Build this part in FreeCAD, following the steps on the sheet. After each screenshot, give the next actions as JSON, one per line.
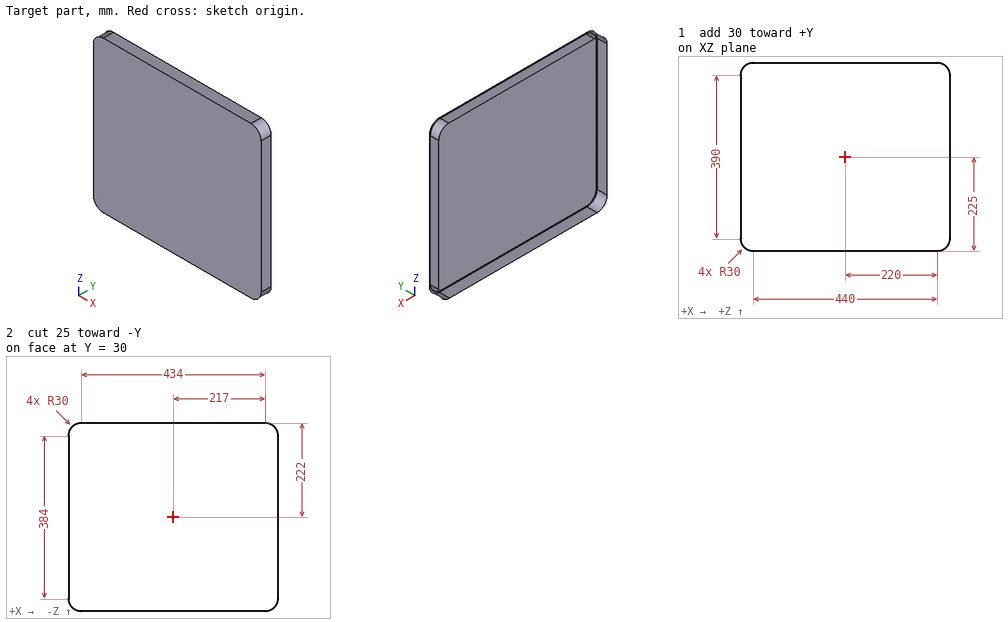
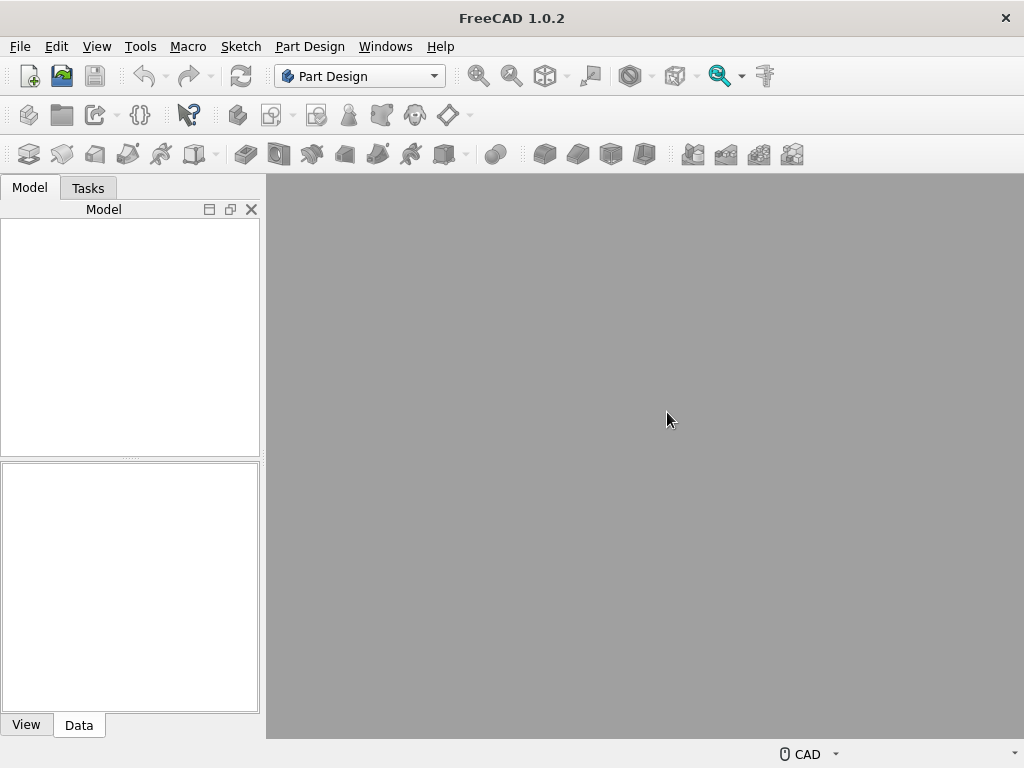
{"action": "left_click", "coordinate": [29, 76]}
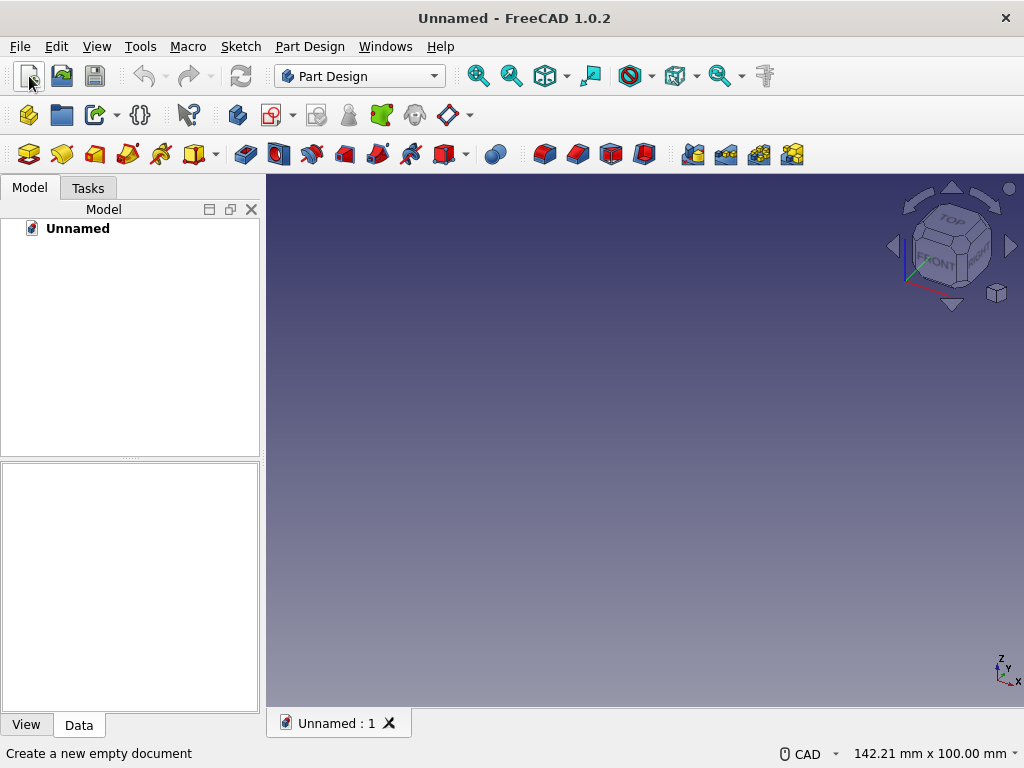
{"action": "left_click", "coordinate": [270, 116]}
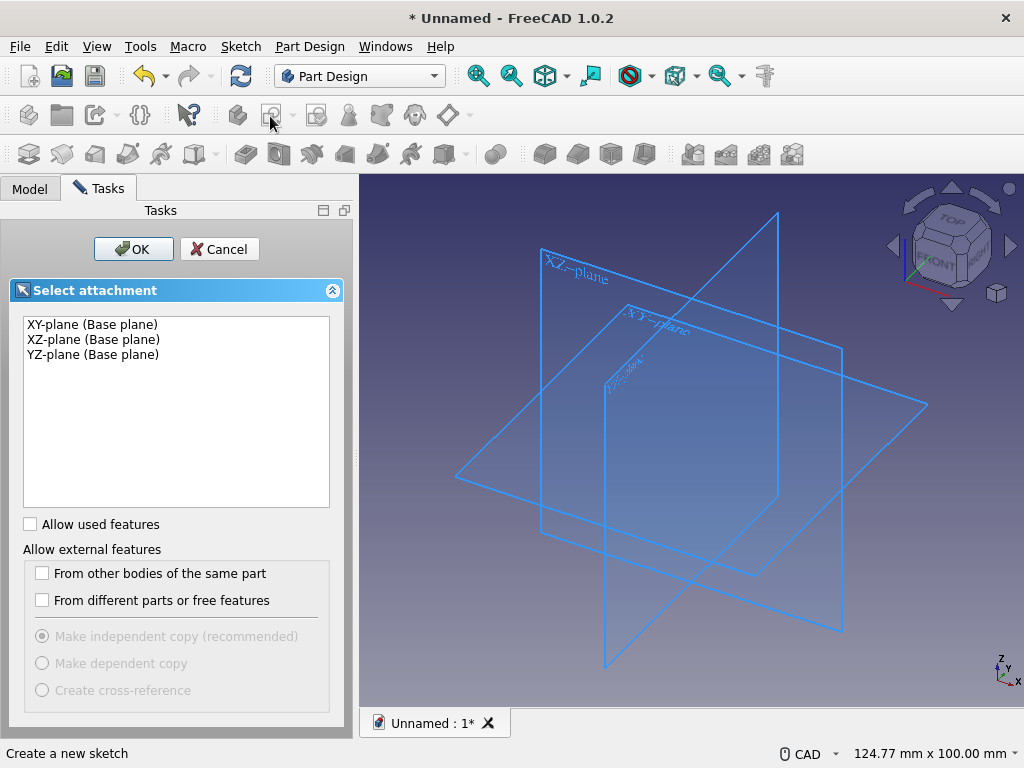
{"action": "left_click", "coordinate": [84, 340]}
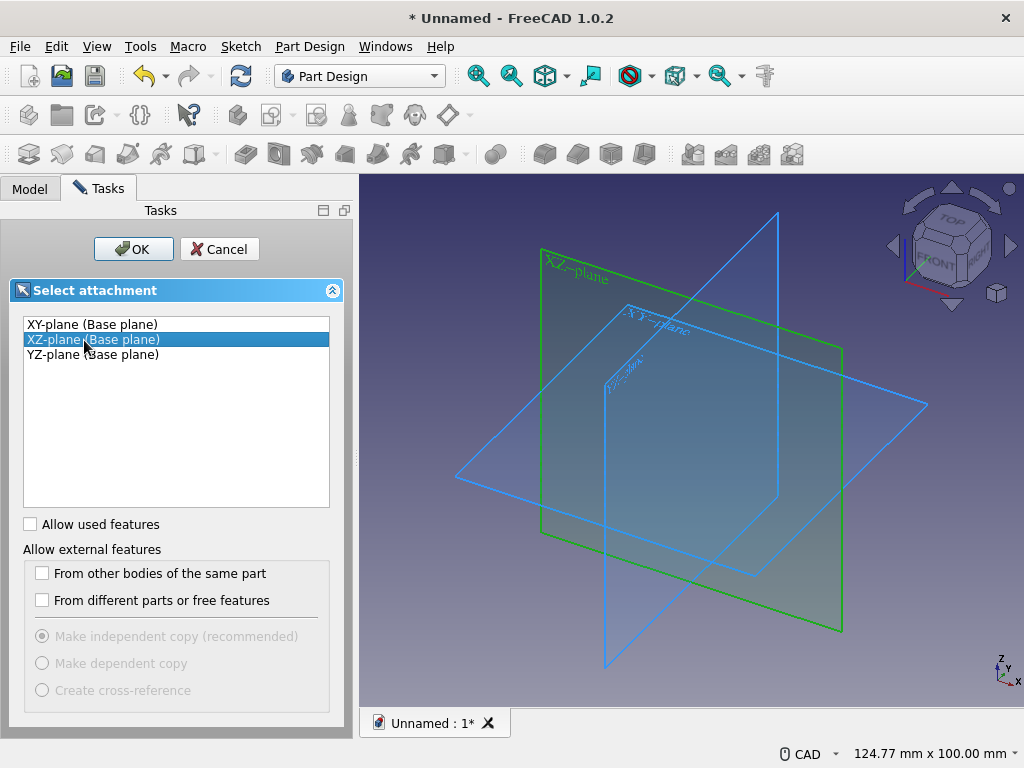
{"action": "left_click", "coordinate": [134, 249]}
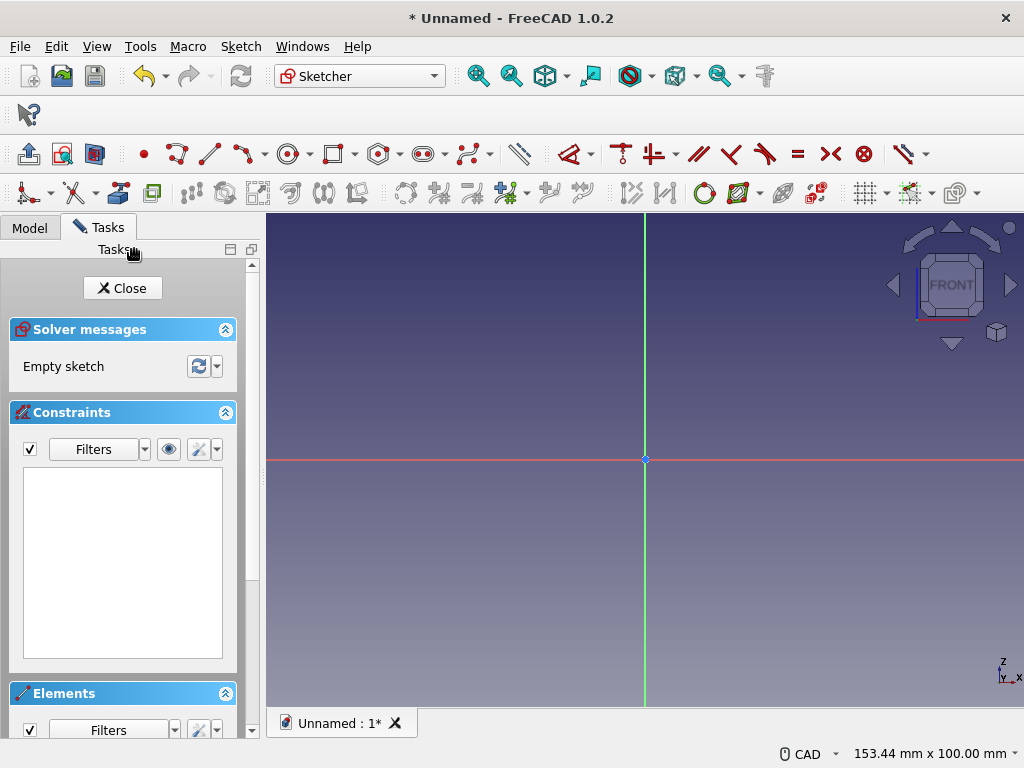
{"action": "scroll", "coordinate": [566, 460], "scroll_direction": "down", "scroll_amount": 10}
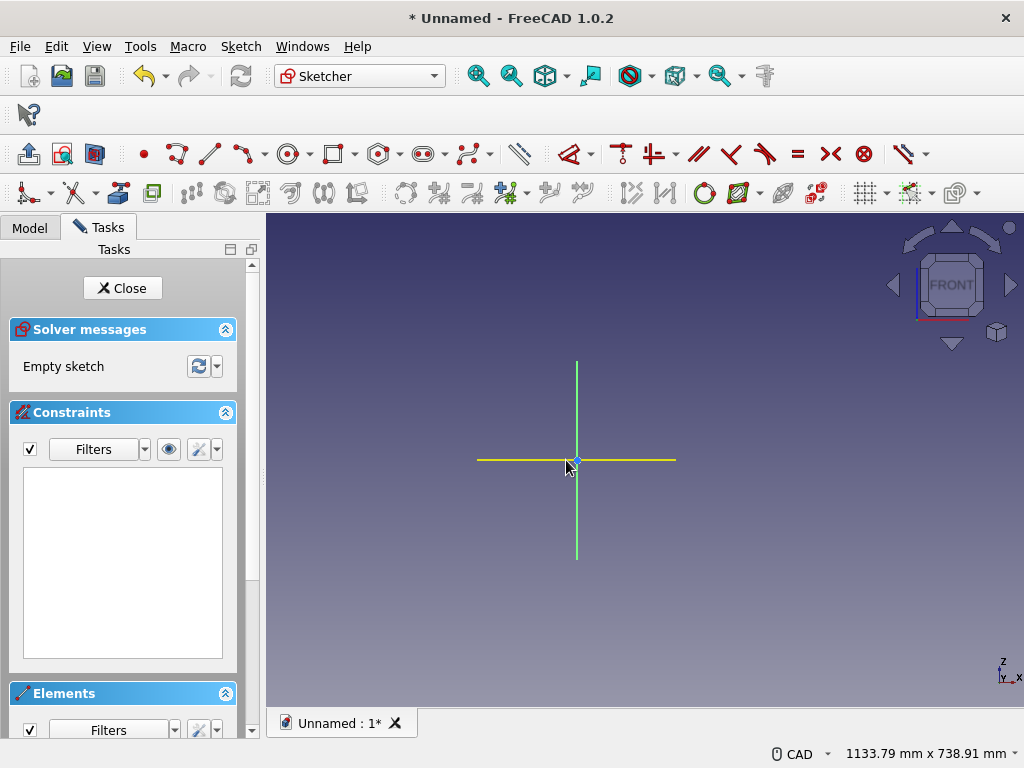
{"action": "left_click", "coordinate": [210, 154]}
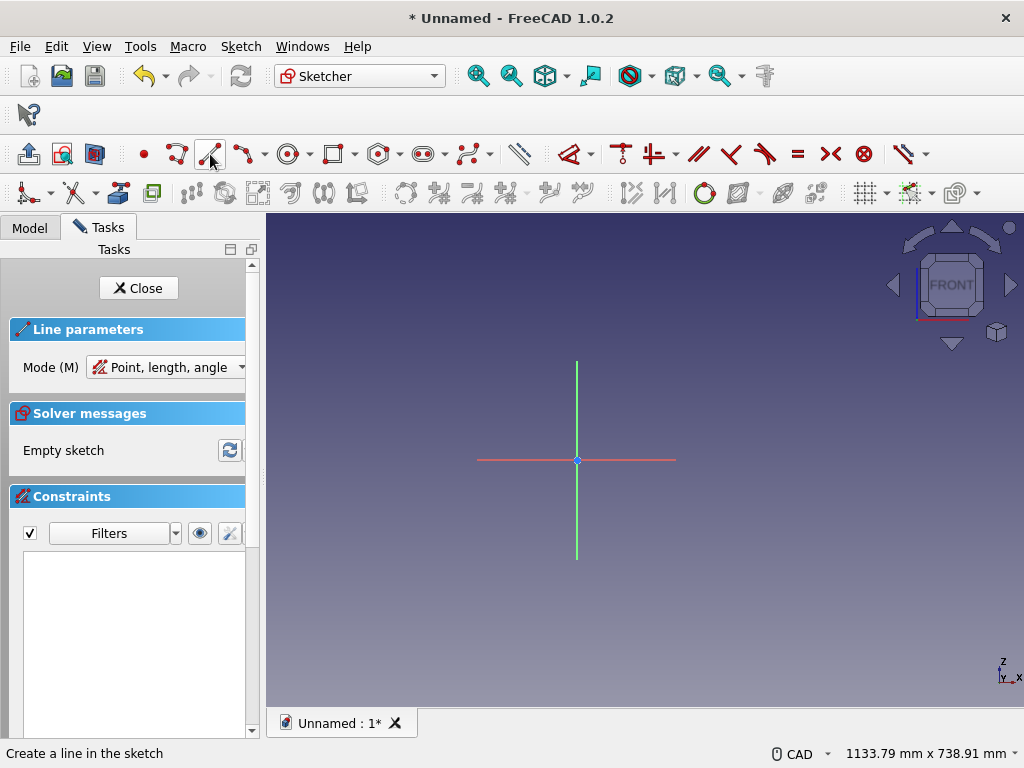
{"action": "left_click", "coordinate": [724, 611]}
{"action": "left_click", "coordinate": [430, 611]}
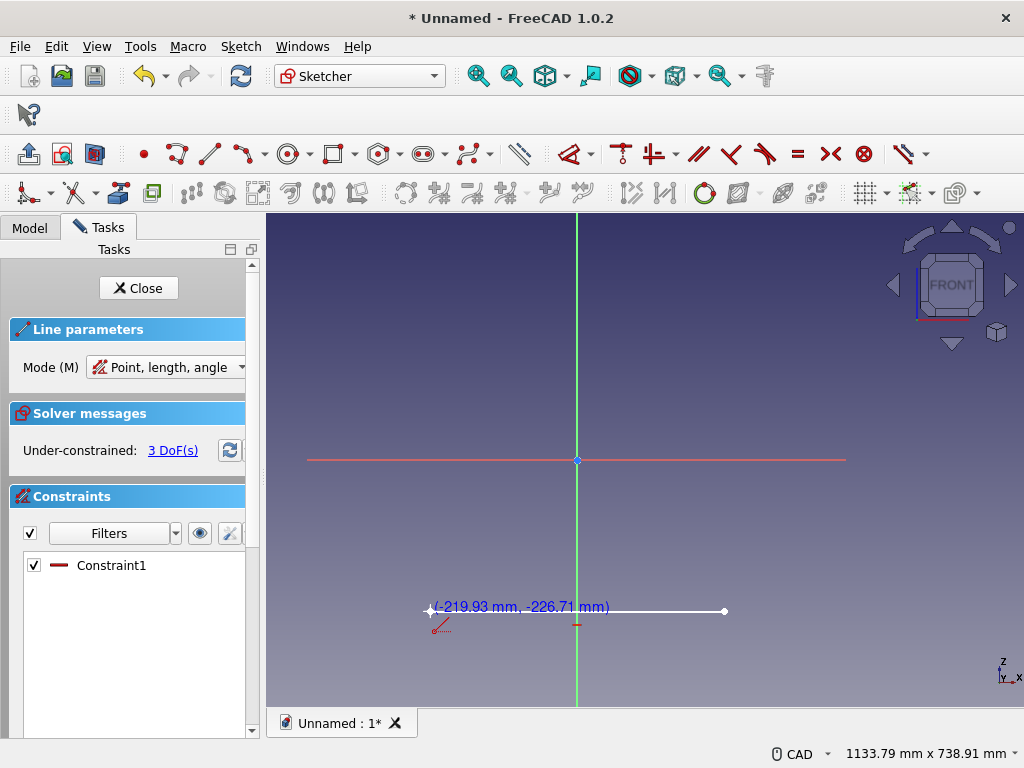
{"action": "left_click", "coordinate": [410, 591]}
{"action": "left_click", "coordinate": [410, 330]}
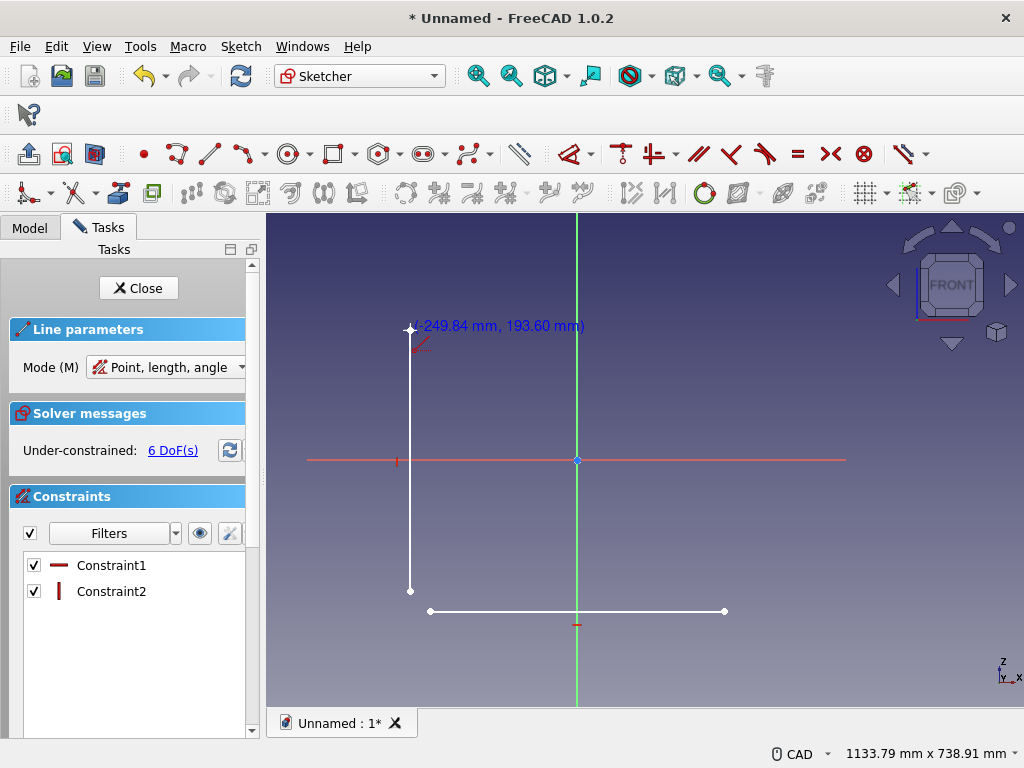
{"action": "left_click", "coordinate": [430, 310]}
{"action": "left_click", "coordinate": [724, 310]}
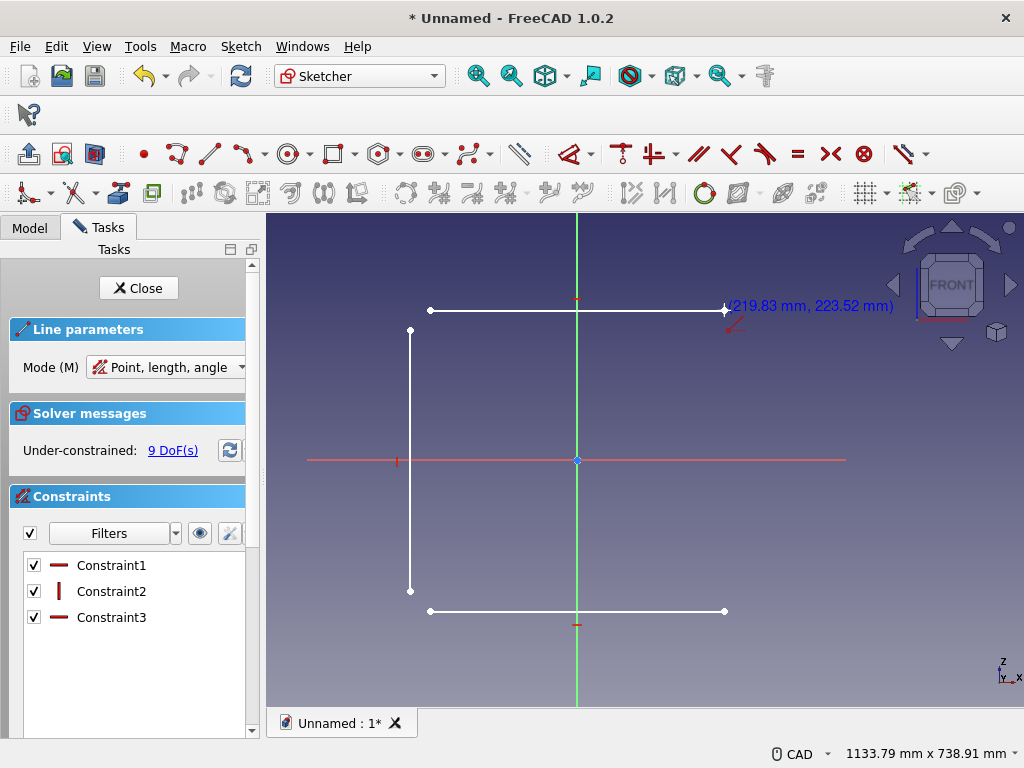
{"action": "left_click", "coordinate": [744, 330]}
{"action": "left_click", "coordinate": [744, 591]}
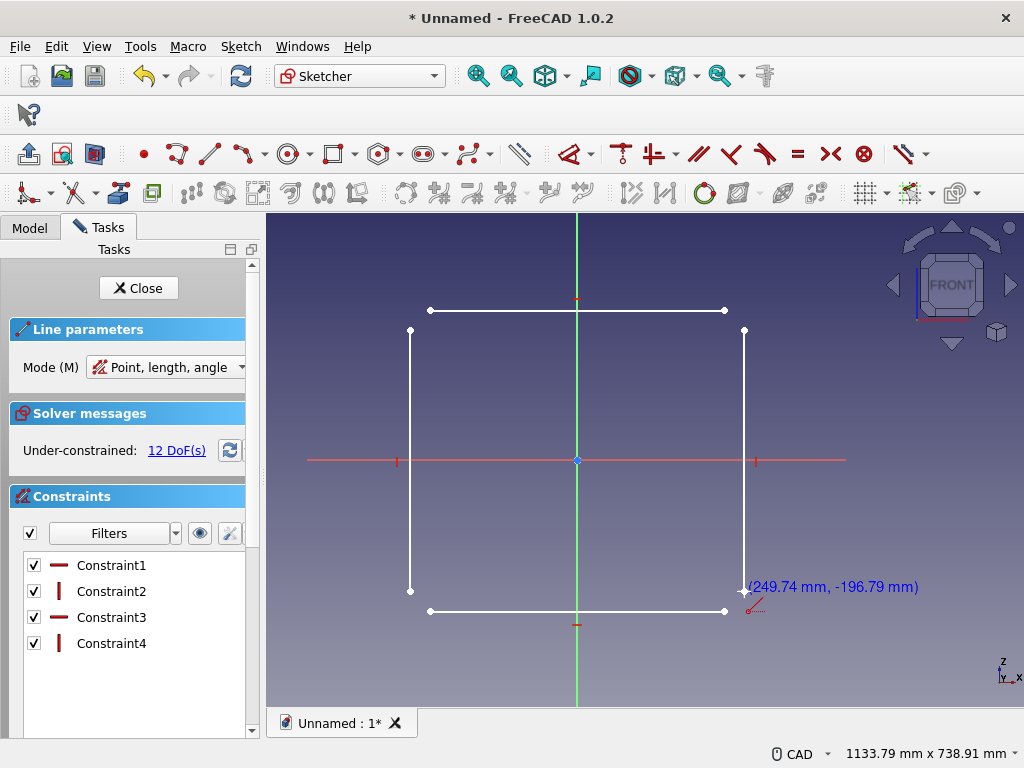
{"action": "left_click", "coordinate": [242, 154]}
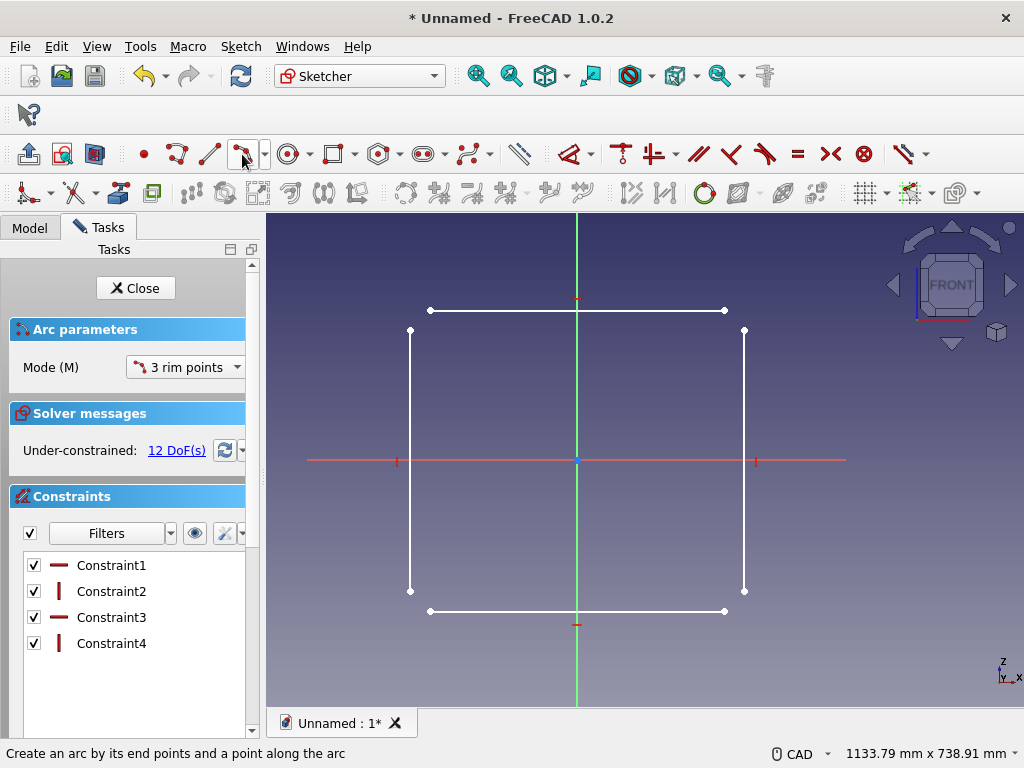
{"action": "left_click", "coordinate": [430, 612]}
{"action": "left_click", "coordinate": [410, 592]}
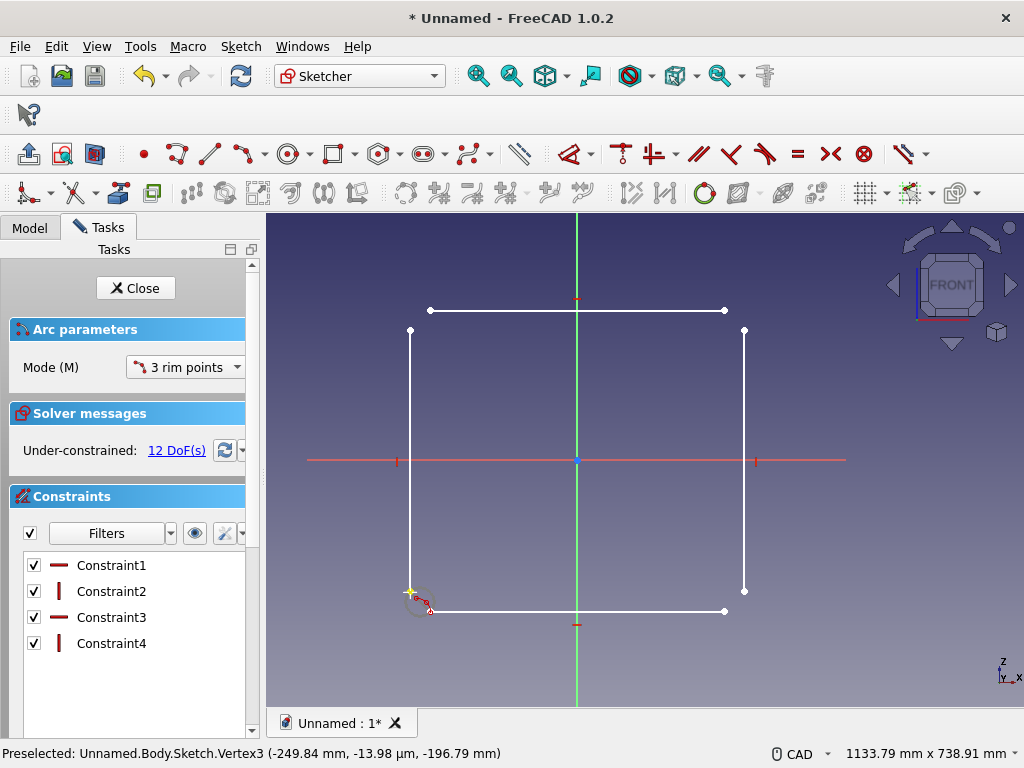
{"action": "scroll", "coordinate": [416, 605], "scroll_direction": "up", "scroll_amount": 5}